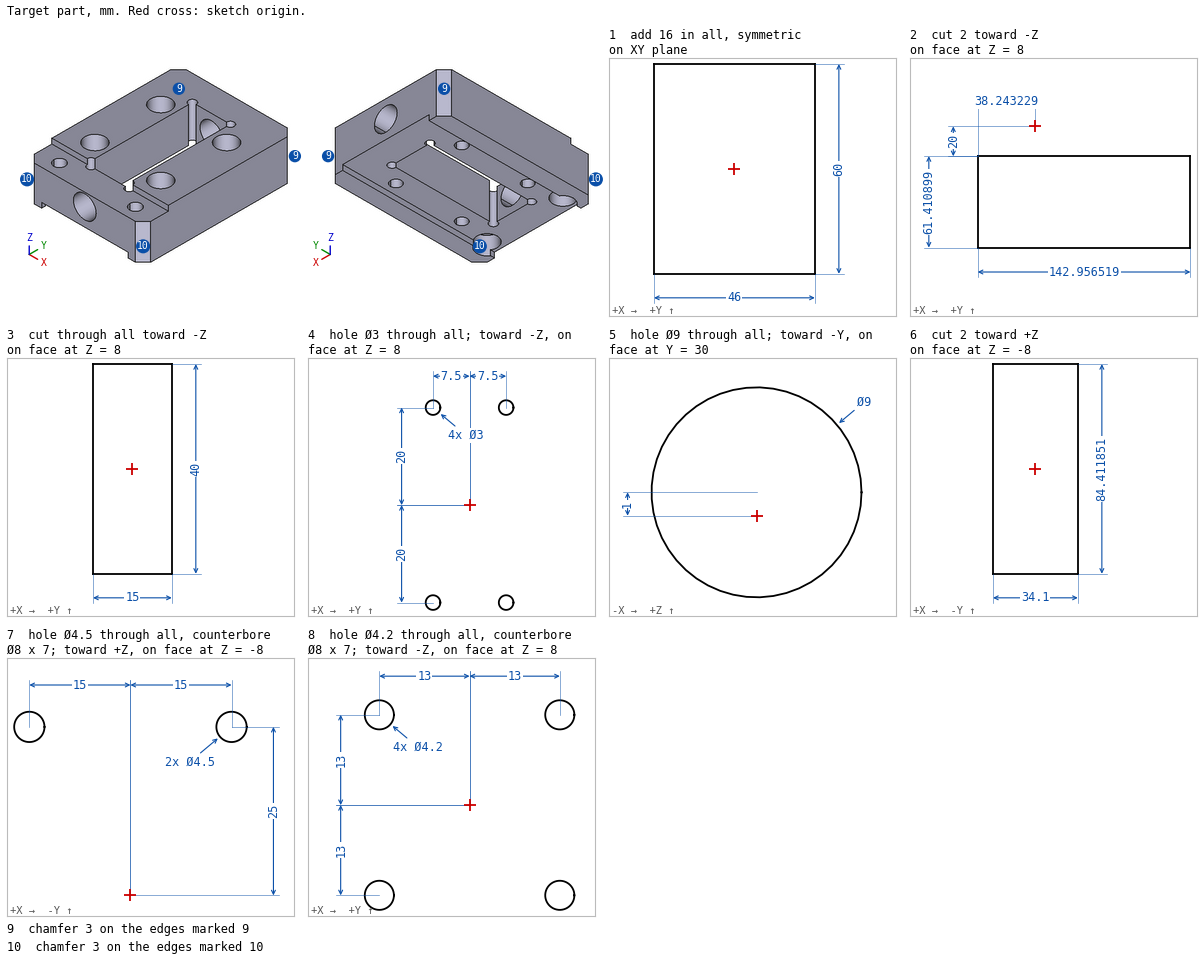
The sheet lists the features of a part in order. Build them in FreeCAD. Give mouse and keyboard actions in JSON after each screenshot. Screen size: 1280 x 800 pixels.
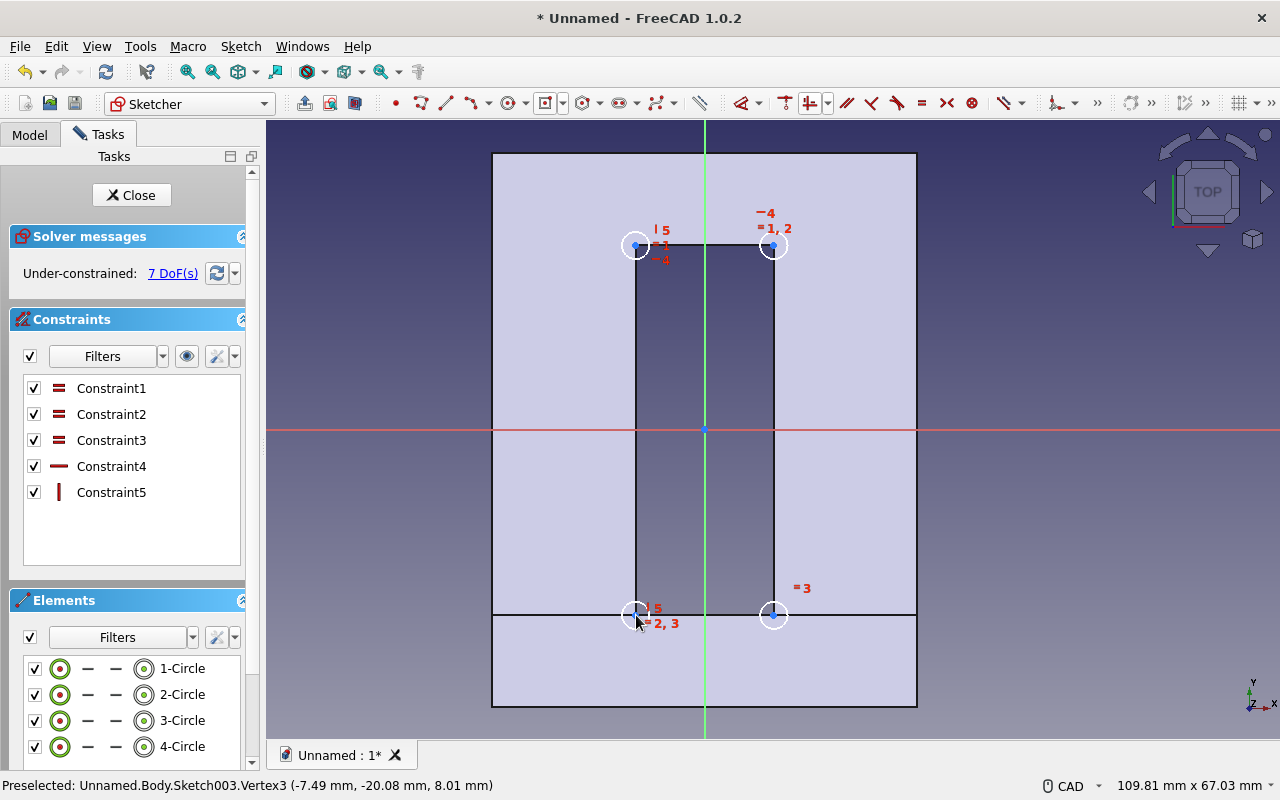
{"action": "left_click", "coordinate": [774, 246]}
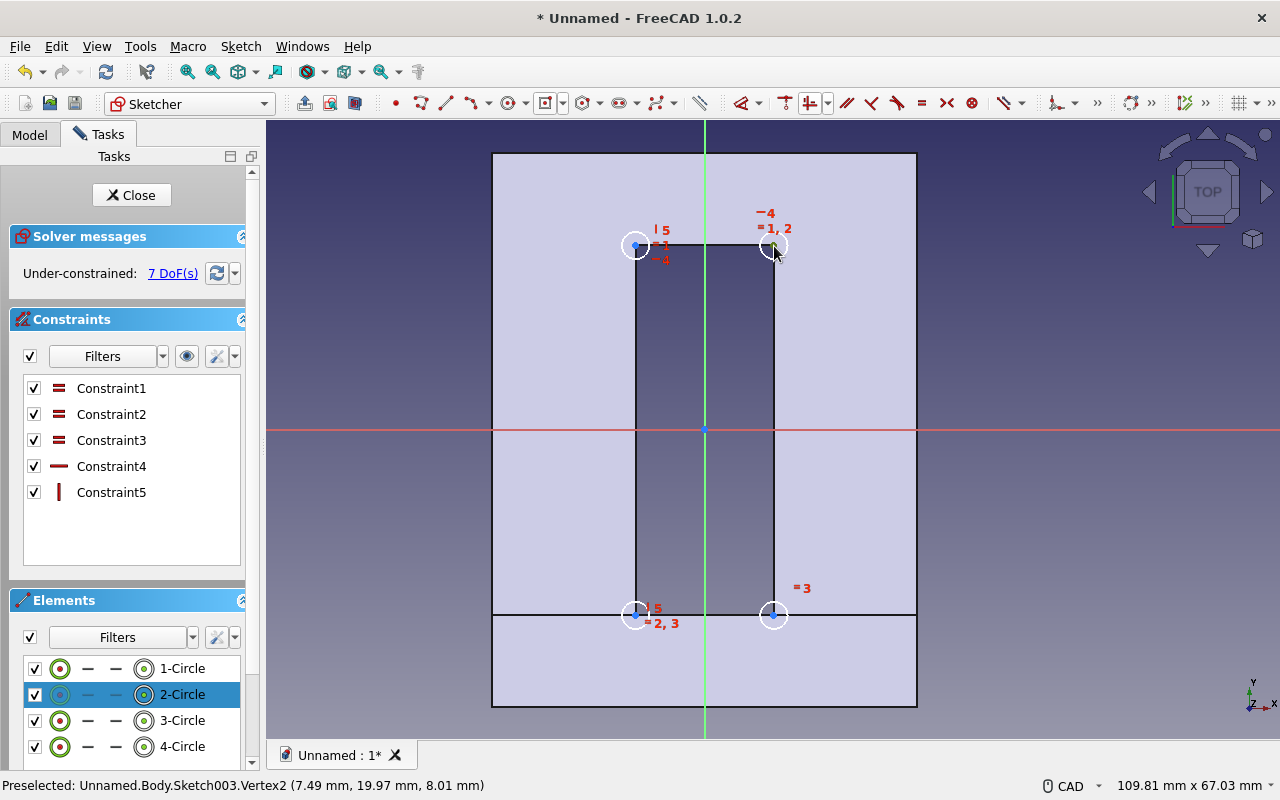
{"action": "left_click", "coordinate": [774, 615]}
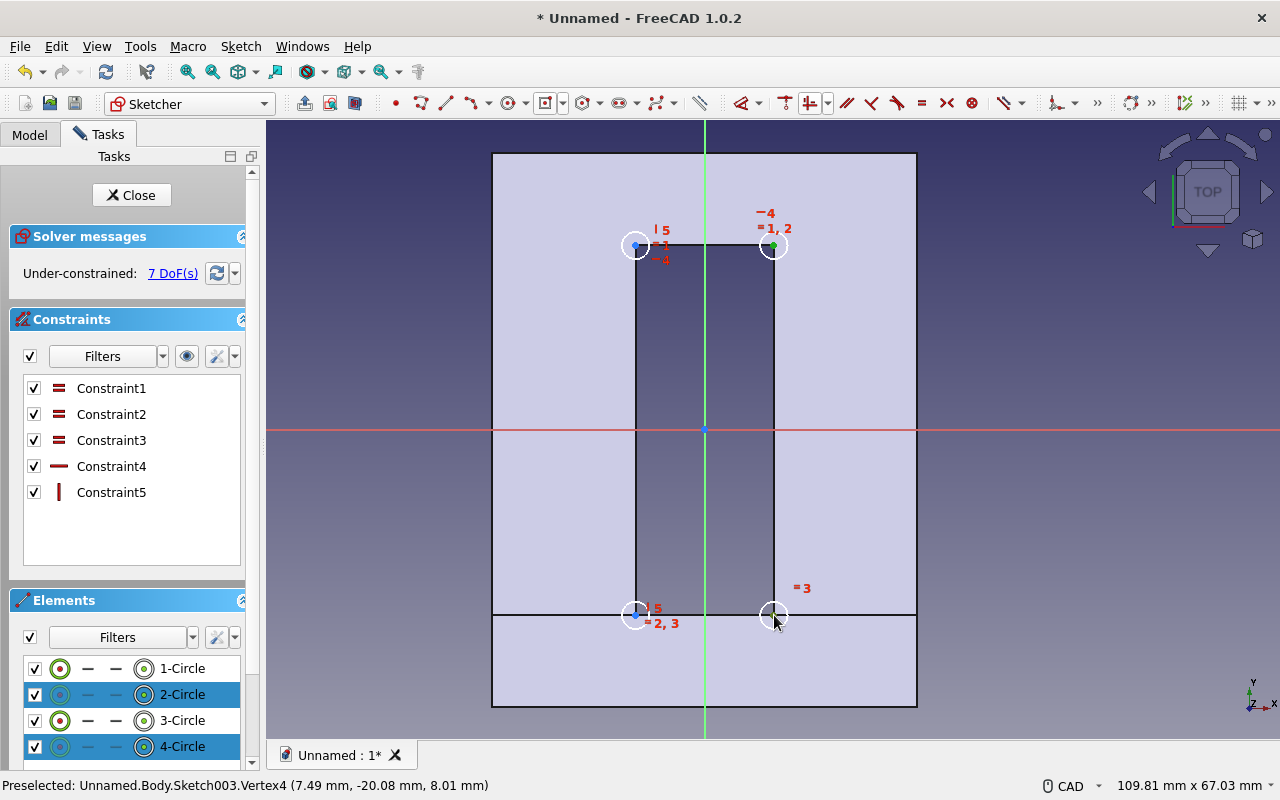
{"action": "key", "text": "v"}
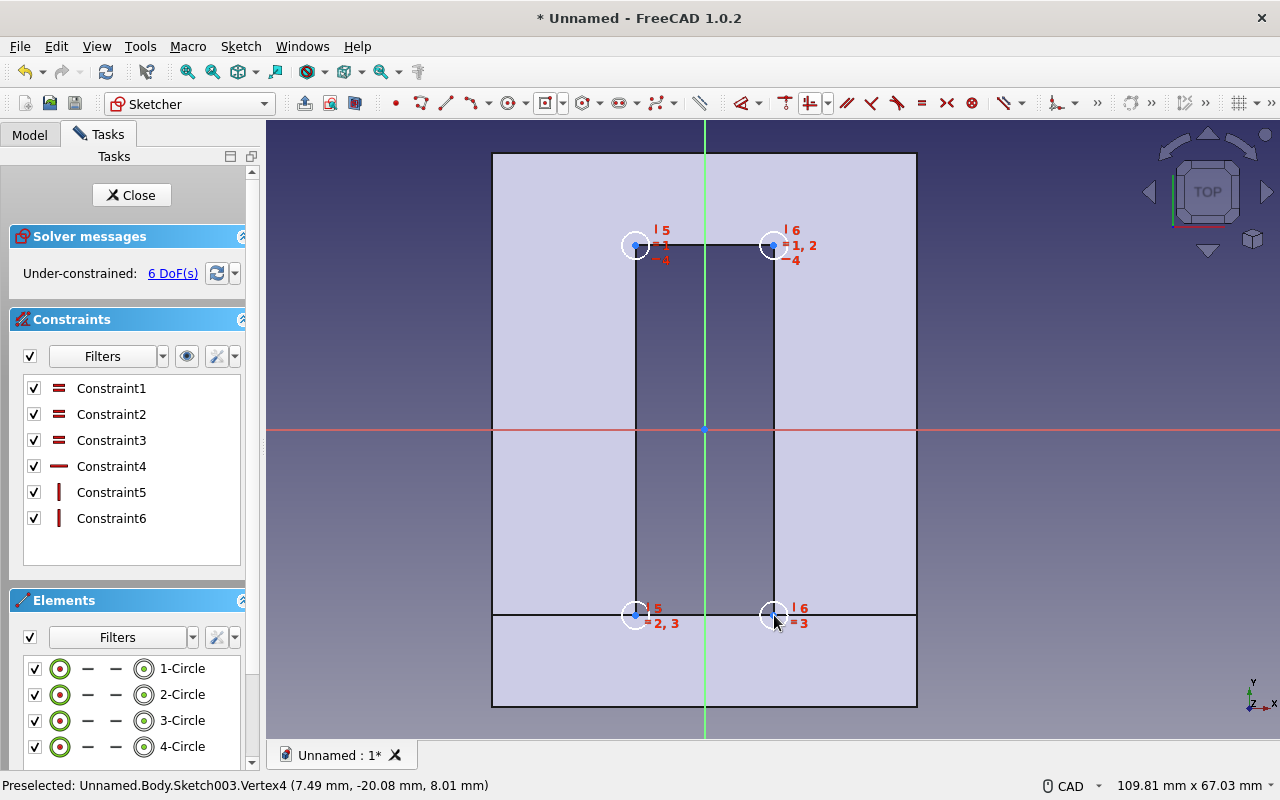
{"action": "left_click", "coordinate": [636, 615]}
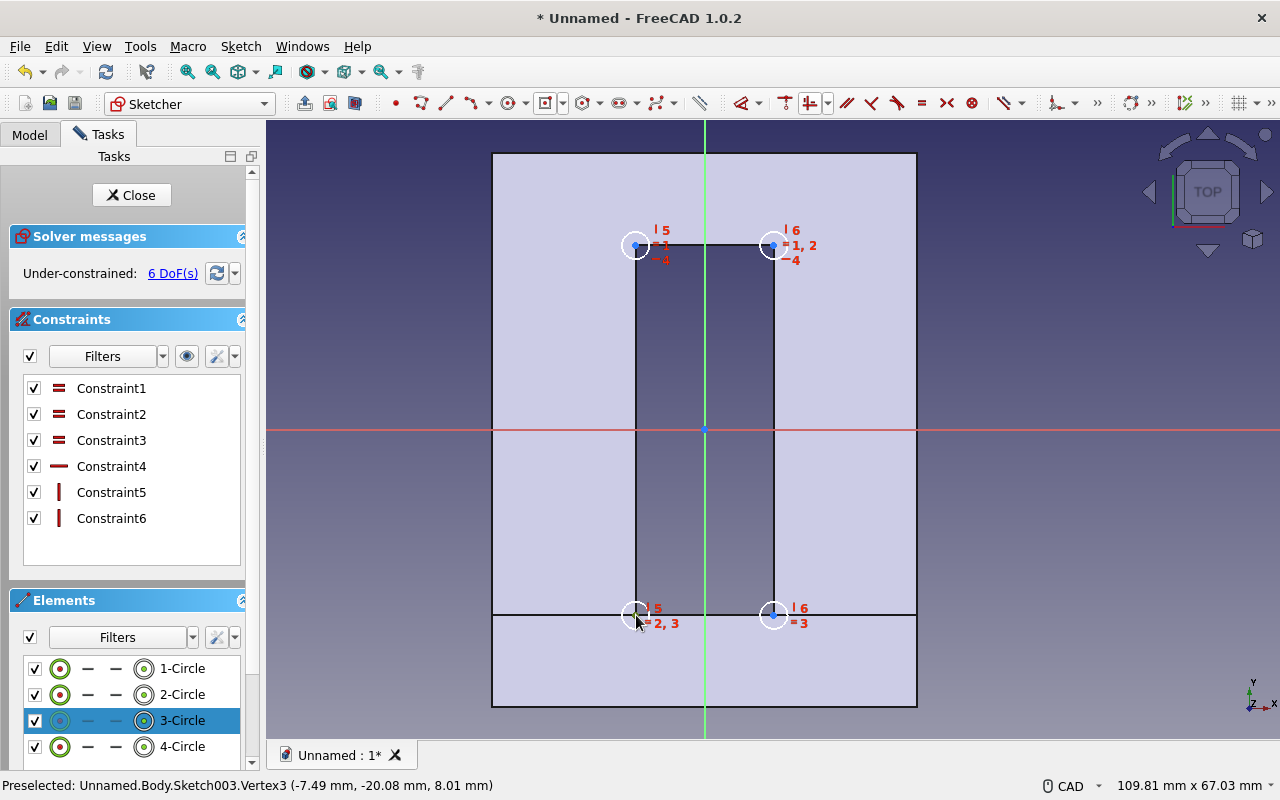
{"action": "left_click", "coordinate": [774, 615]}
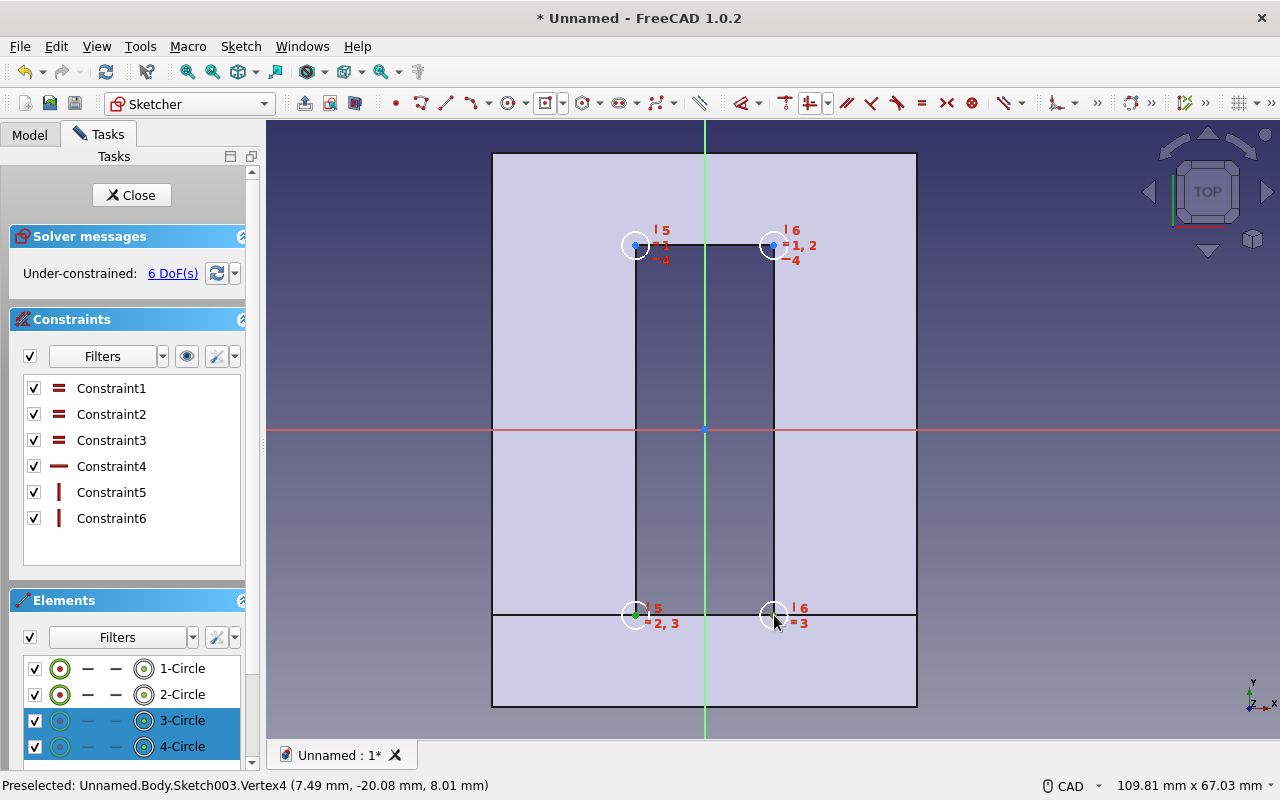
{"action": "left_click", "coordinate": [828, 104]}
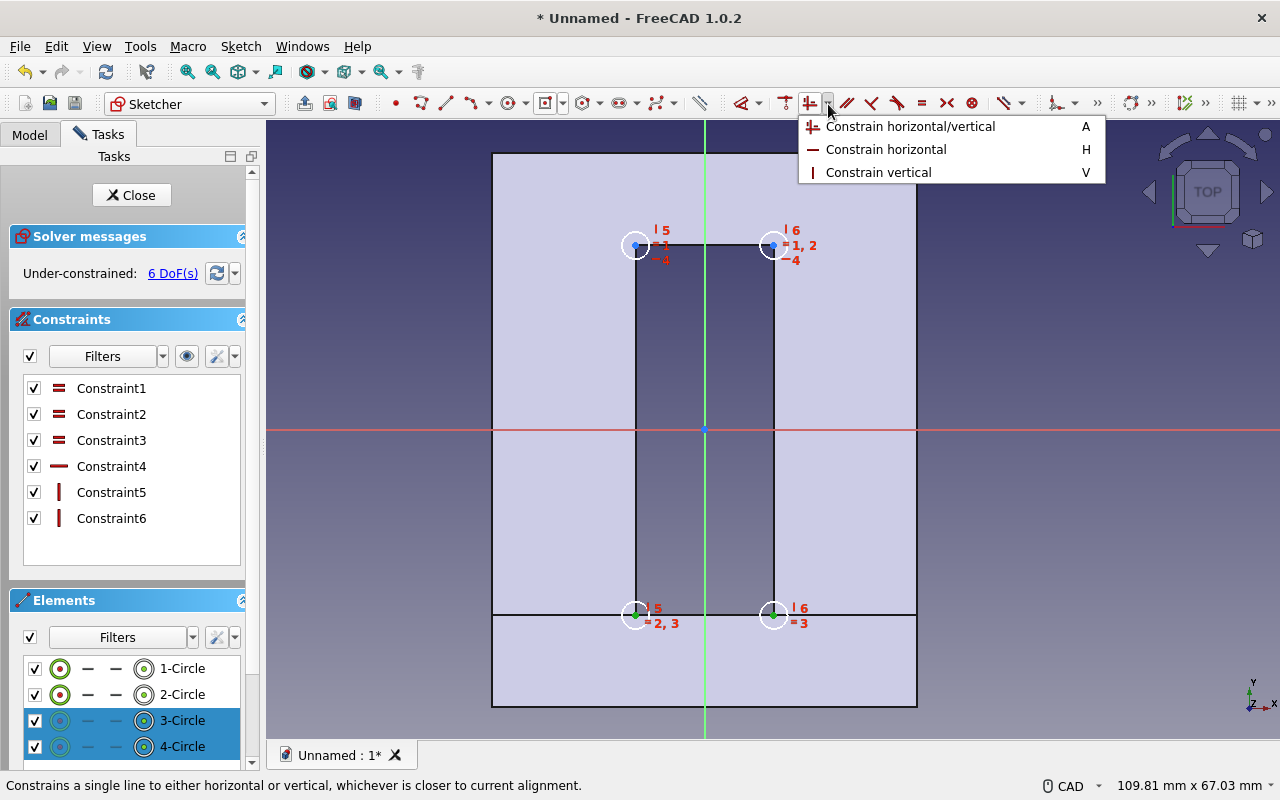
{"action": "left_click", "coordinate": [952, 150]}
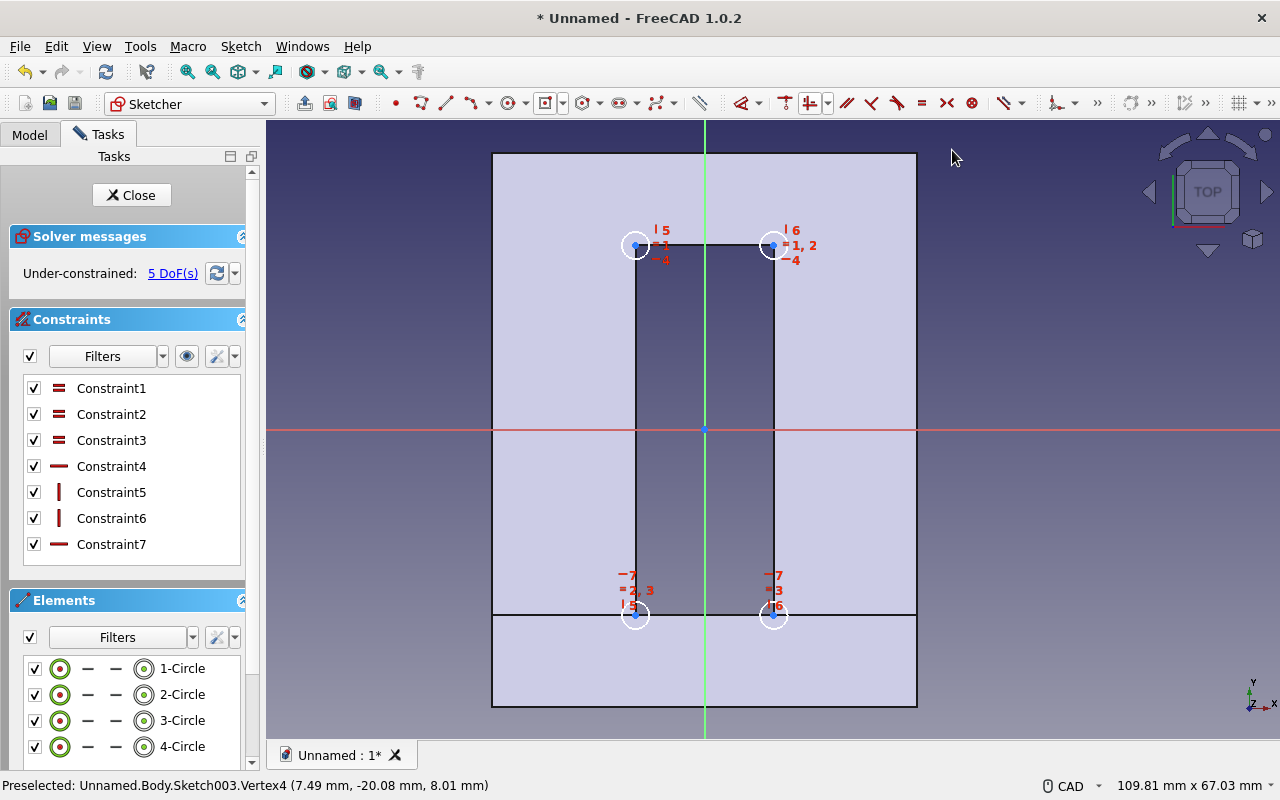
{"action": "left_click", "coordinate": [740, 104]}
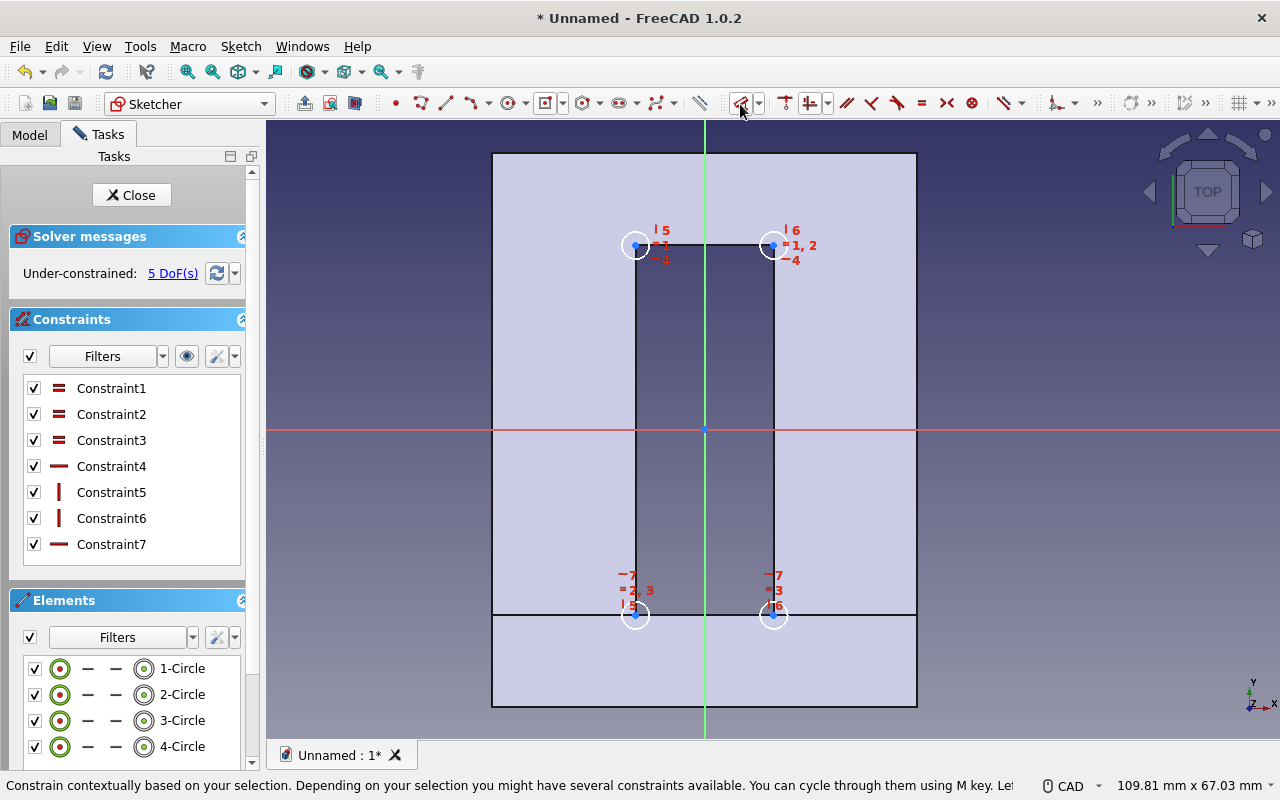
{"action": "scroll", "coordinate": [645, 236], "scroll_direction": "up", "scroll_amount": 2}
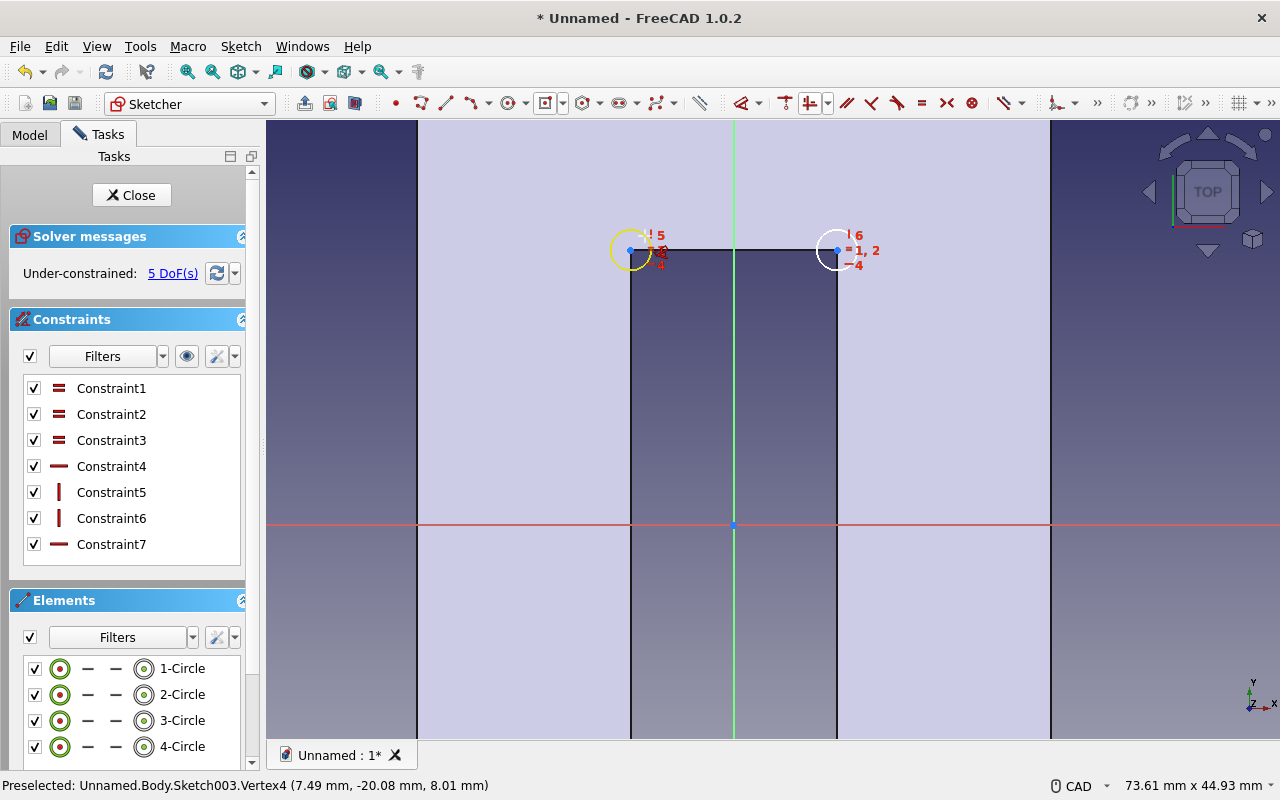
{"action": "left_click", "coordinate": [645, 236]}
{"action": "left_click", "coordinate": [668, 213]}